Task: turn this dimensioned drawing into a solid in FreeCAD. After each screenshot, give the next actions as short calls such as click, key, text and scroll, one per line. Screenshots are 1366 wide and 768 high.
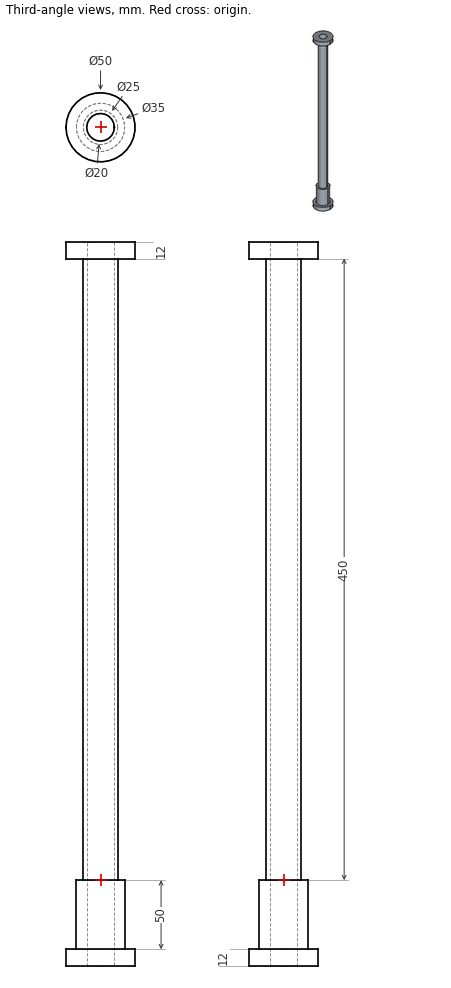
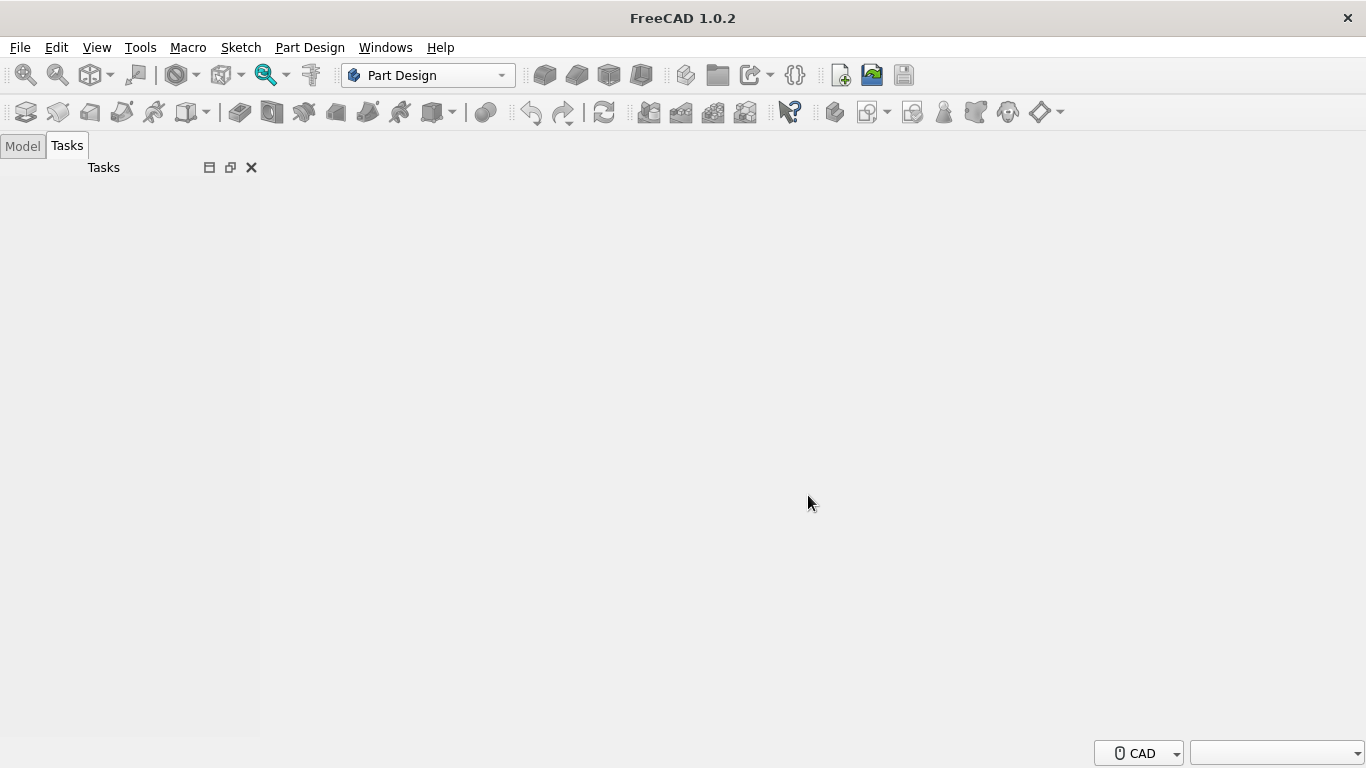
key(ctrl+n)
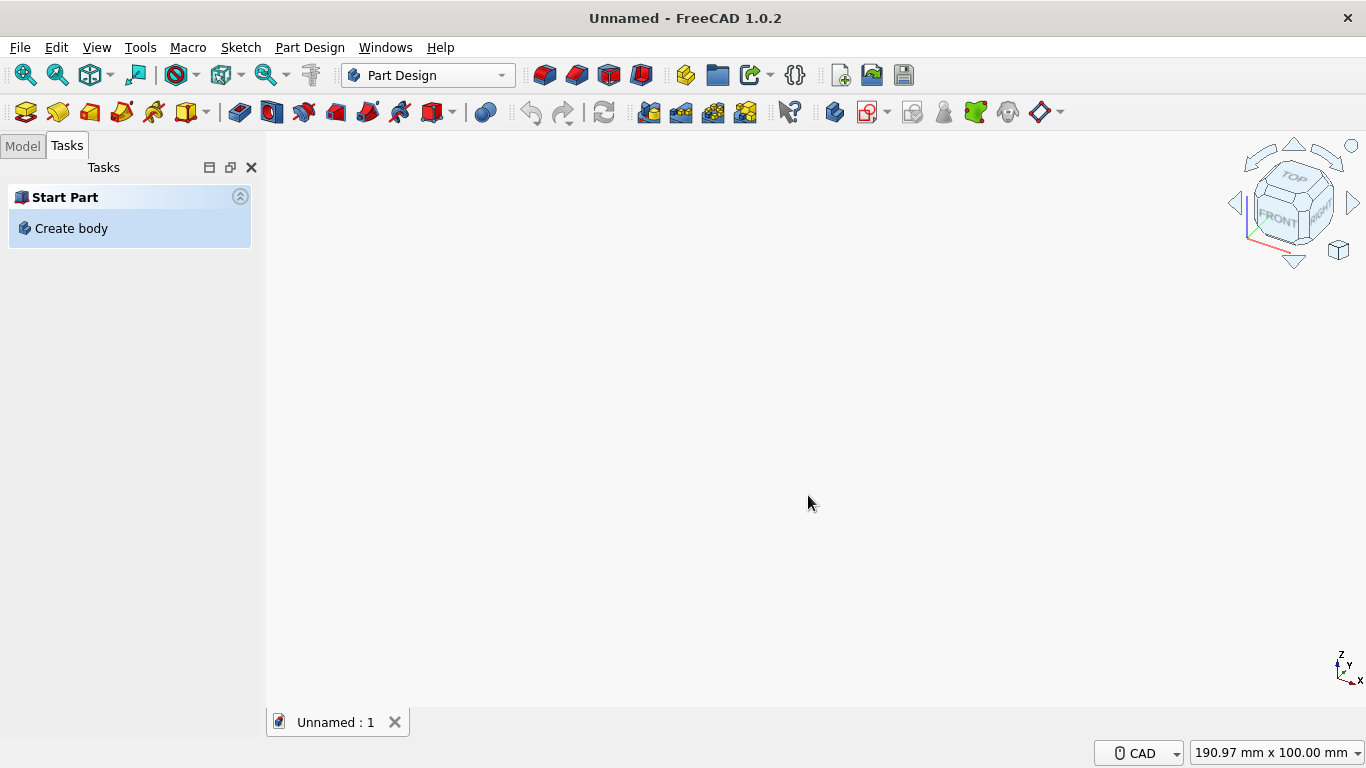
click(868, 112)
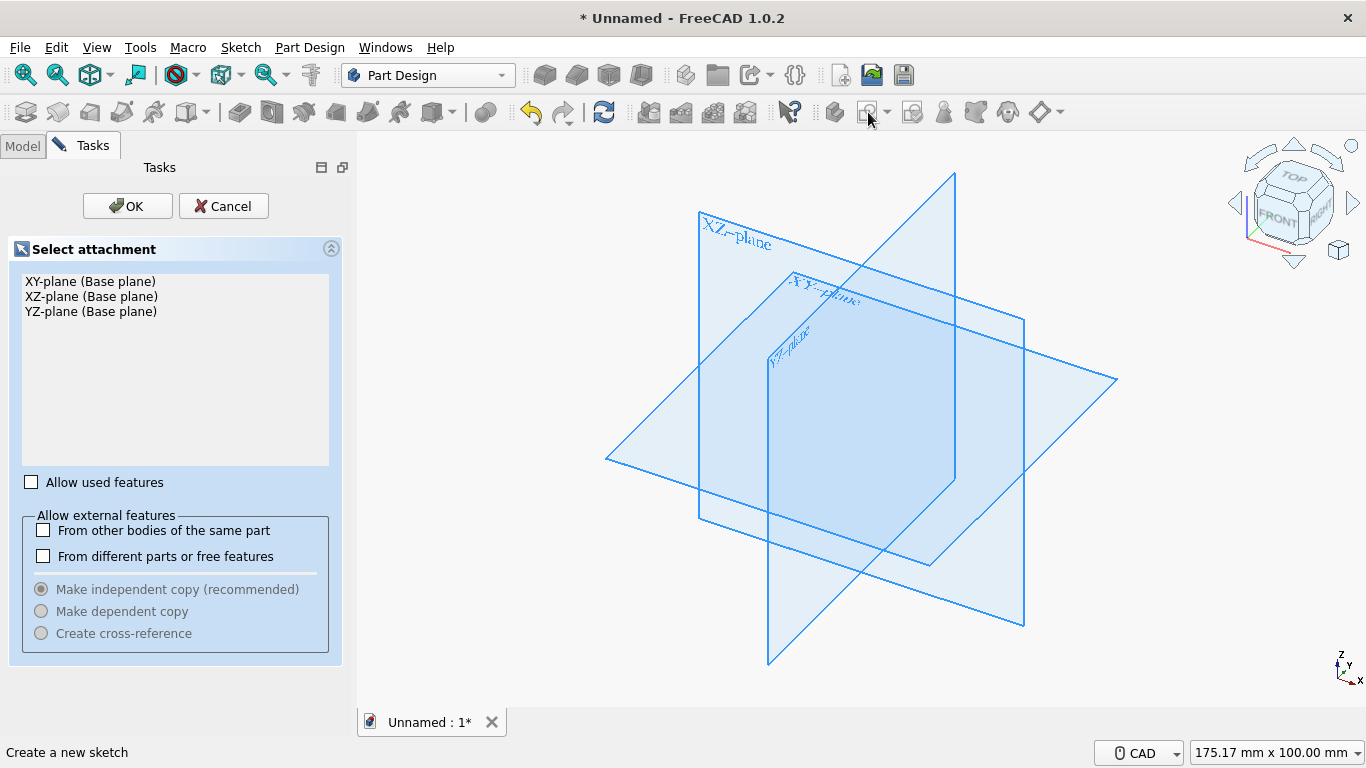
click(82, 282)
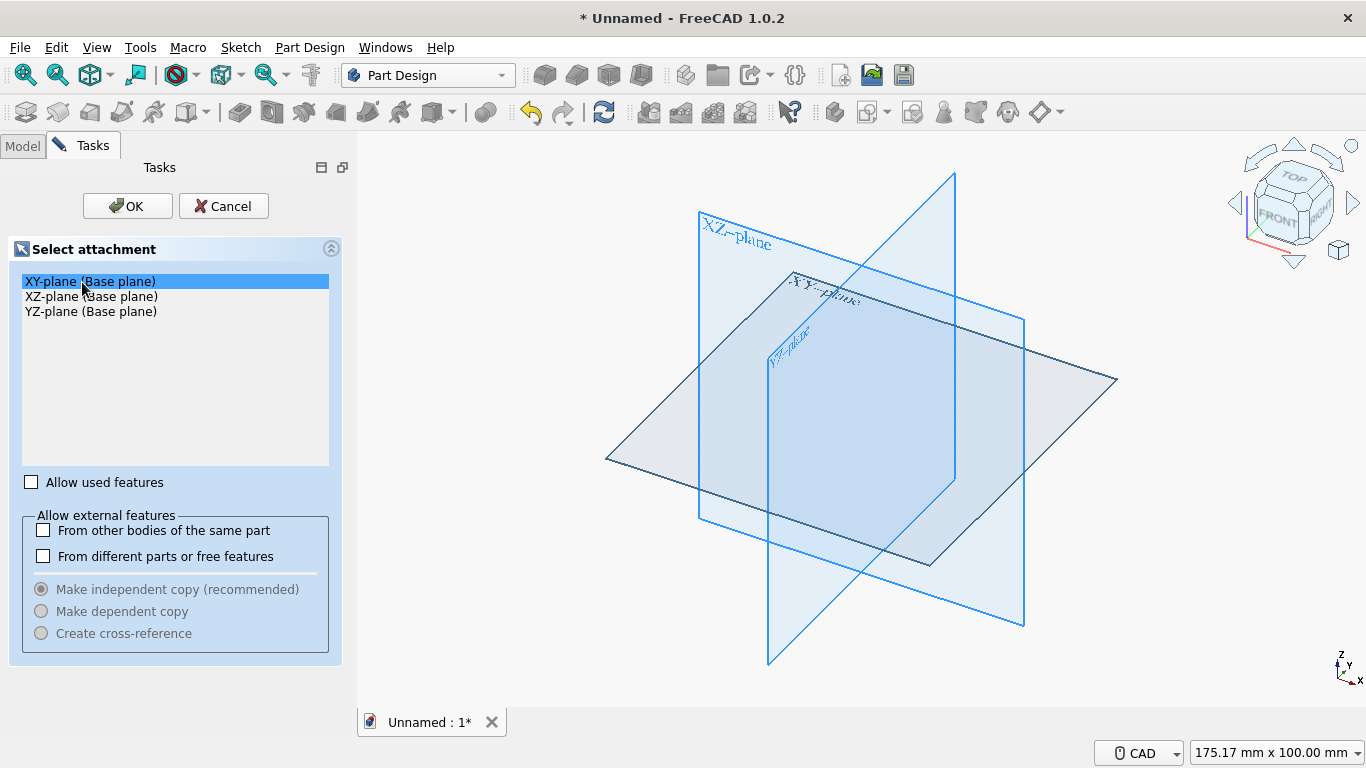
click(128, 206)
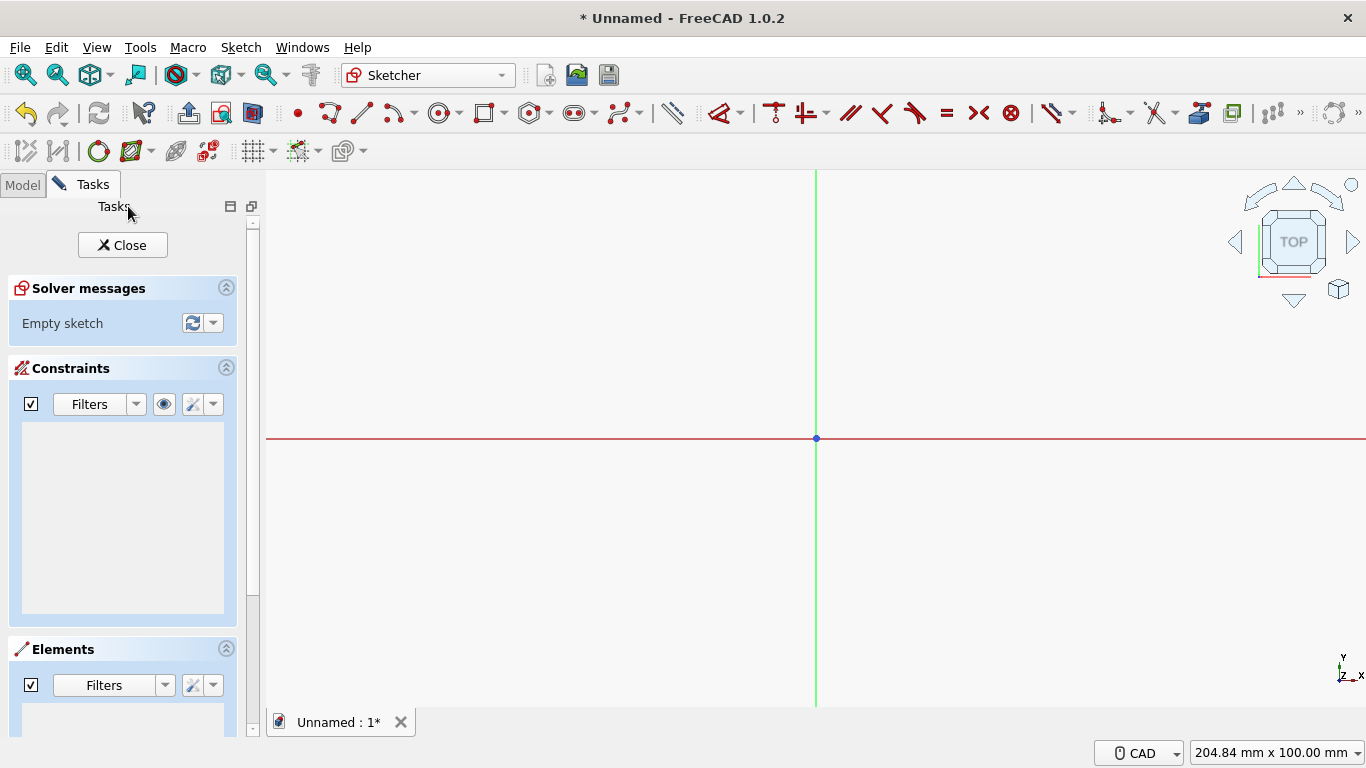
scroll(856, 439, up, 5)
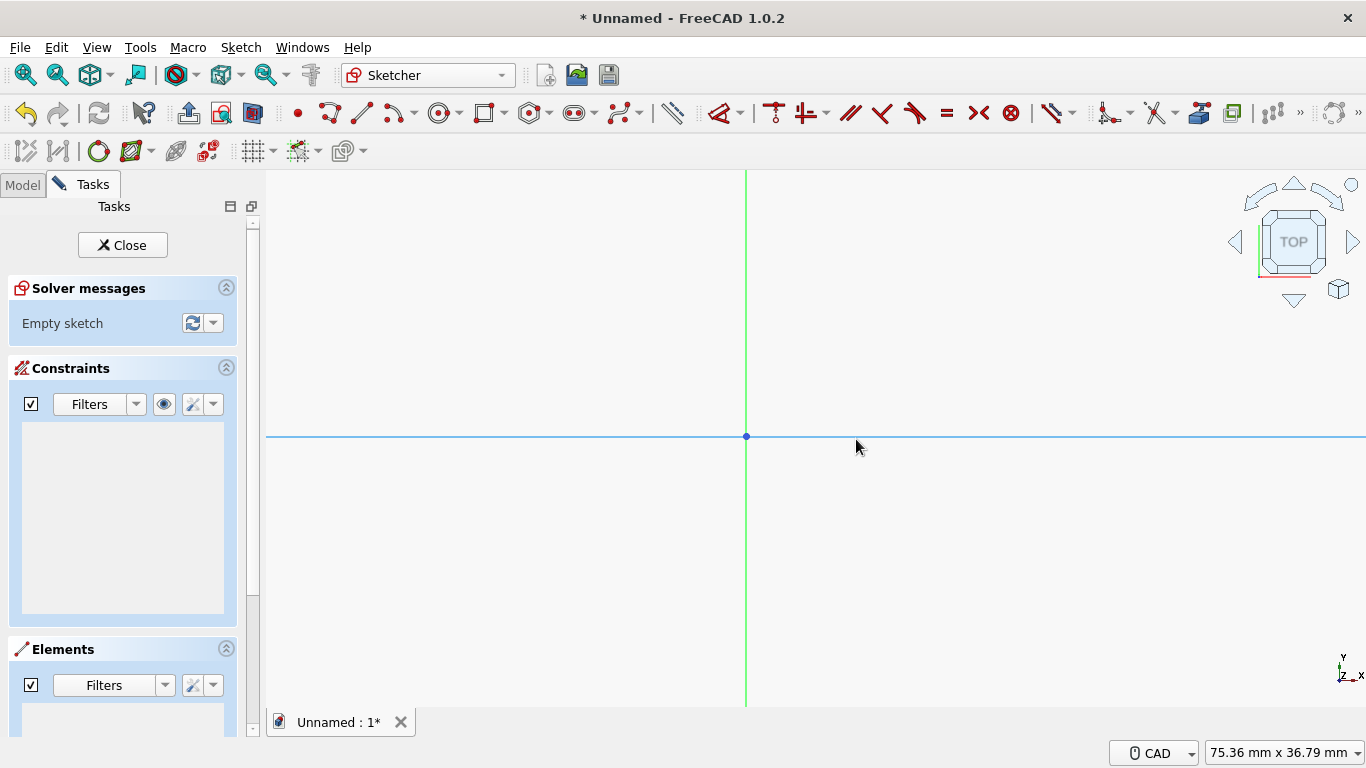
click(440, 114)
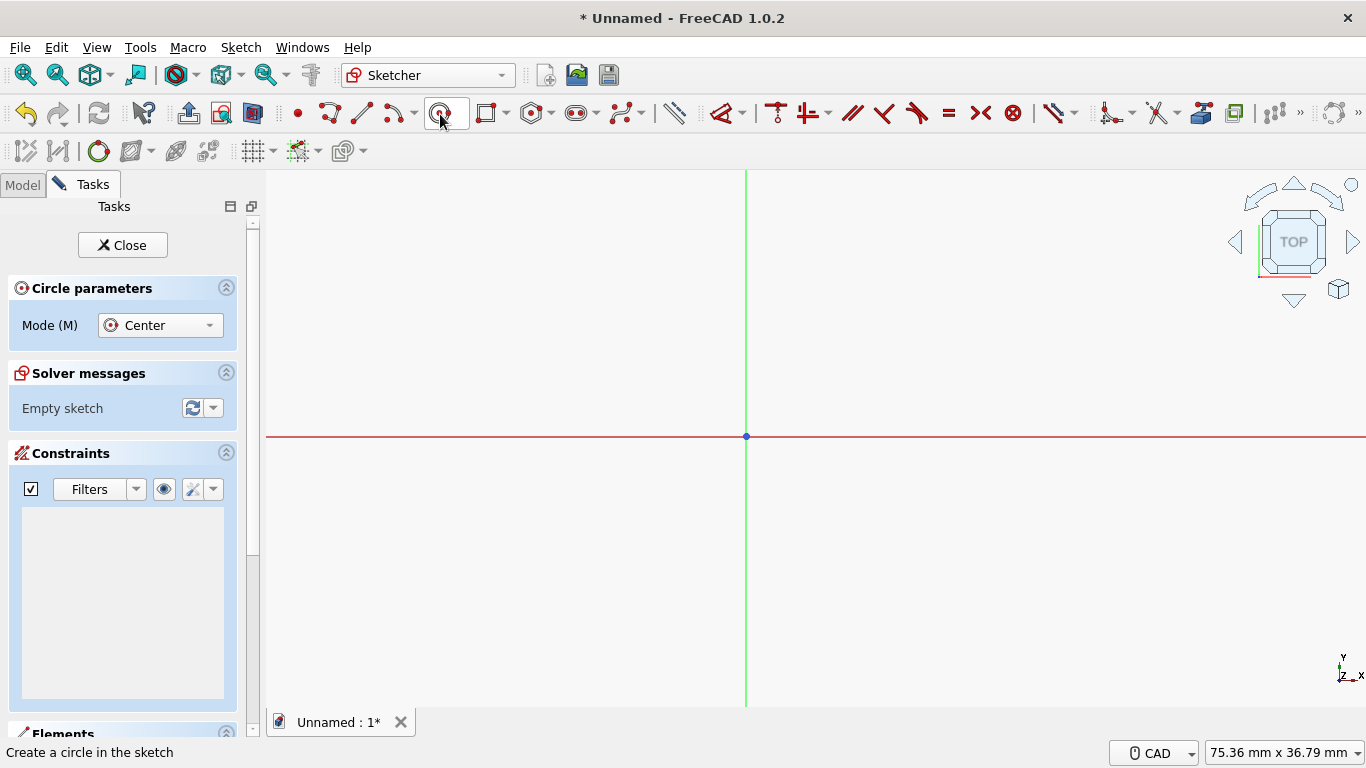
click(746, 437)
click(875, 308)
key(Escape)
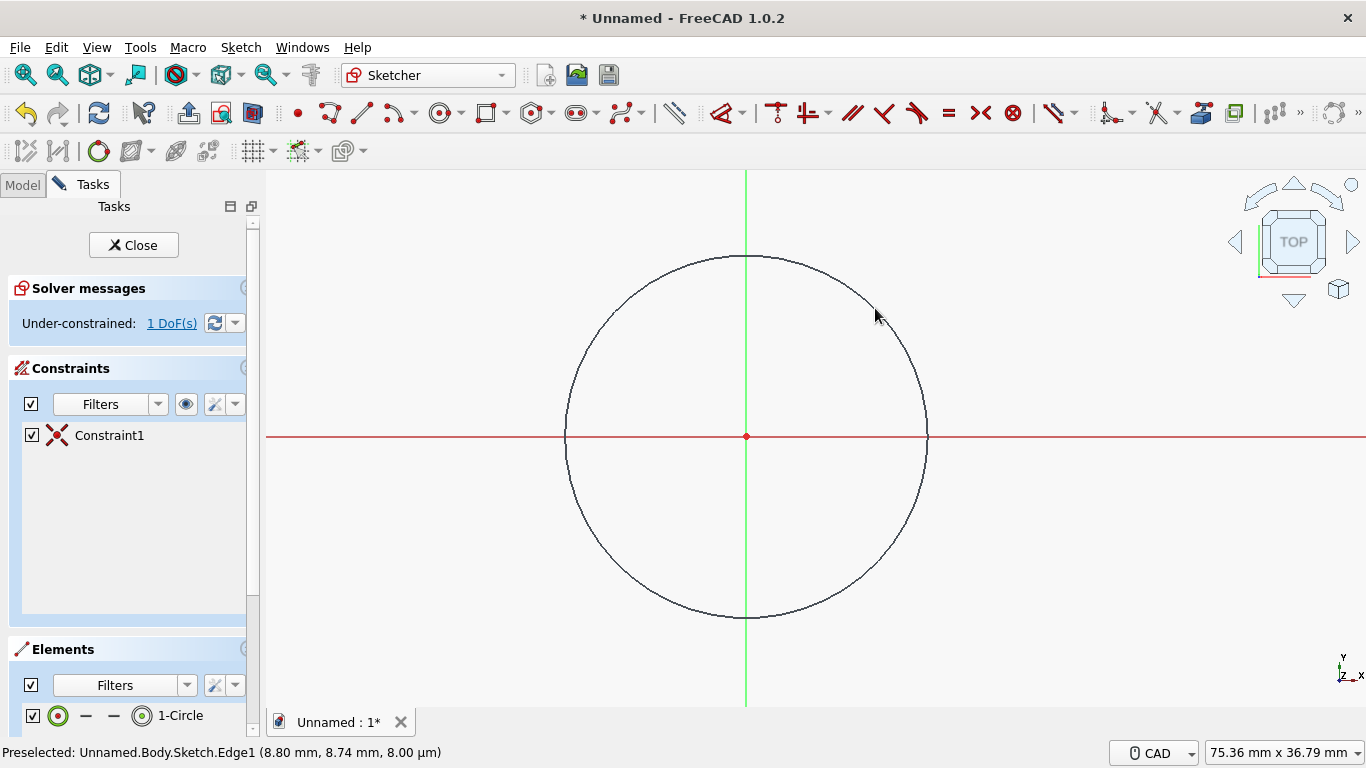
key(d)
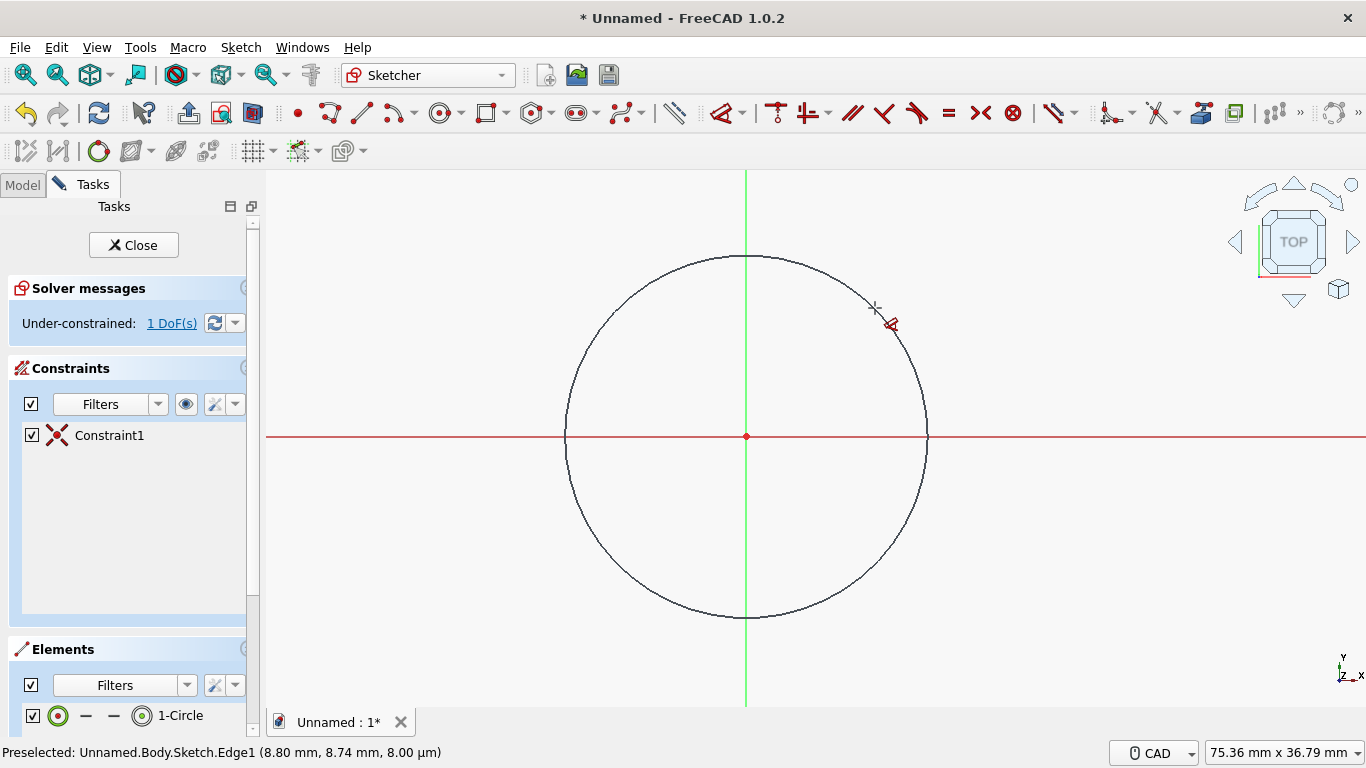
click(874, 308)
click(897, 285)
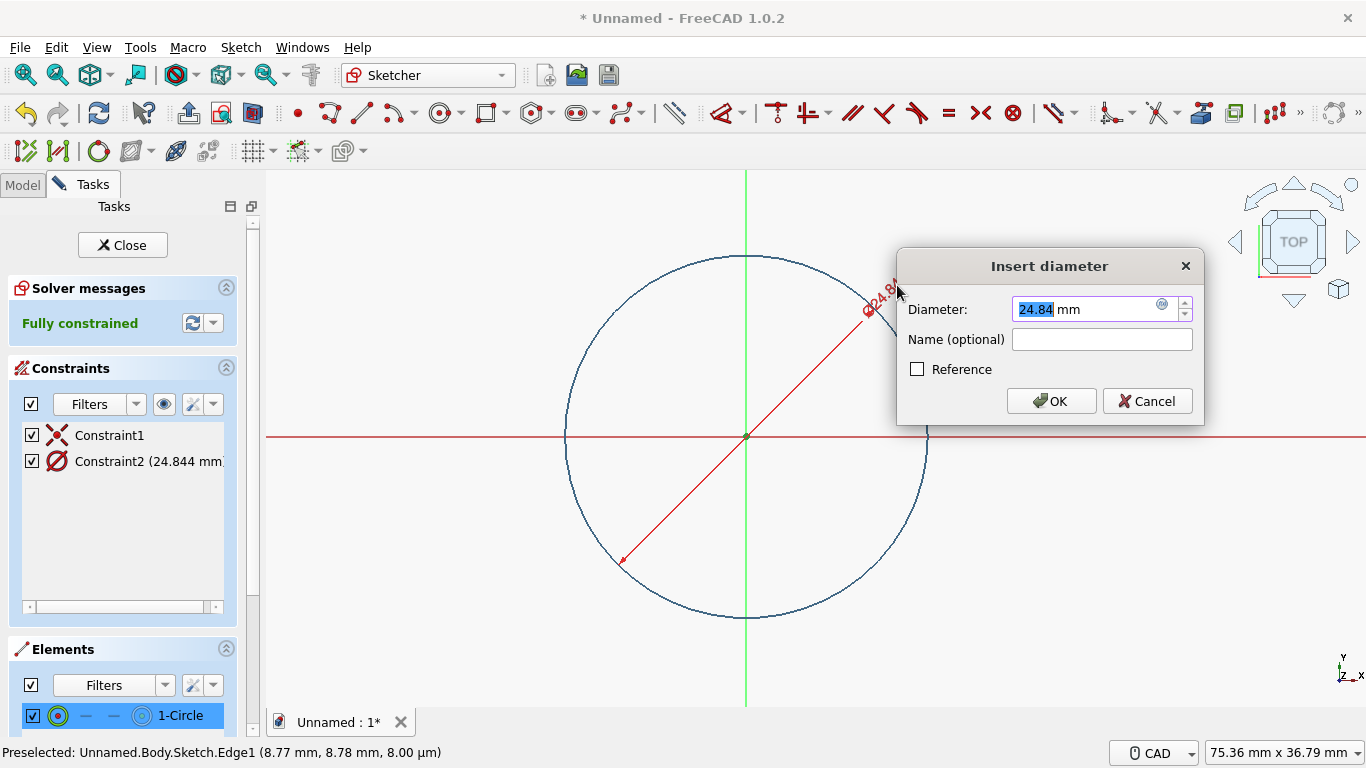
text(25)
key(Return)
key(Escape)